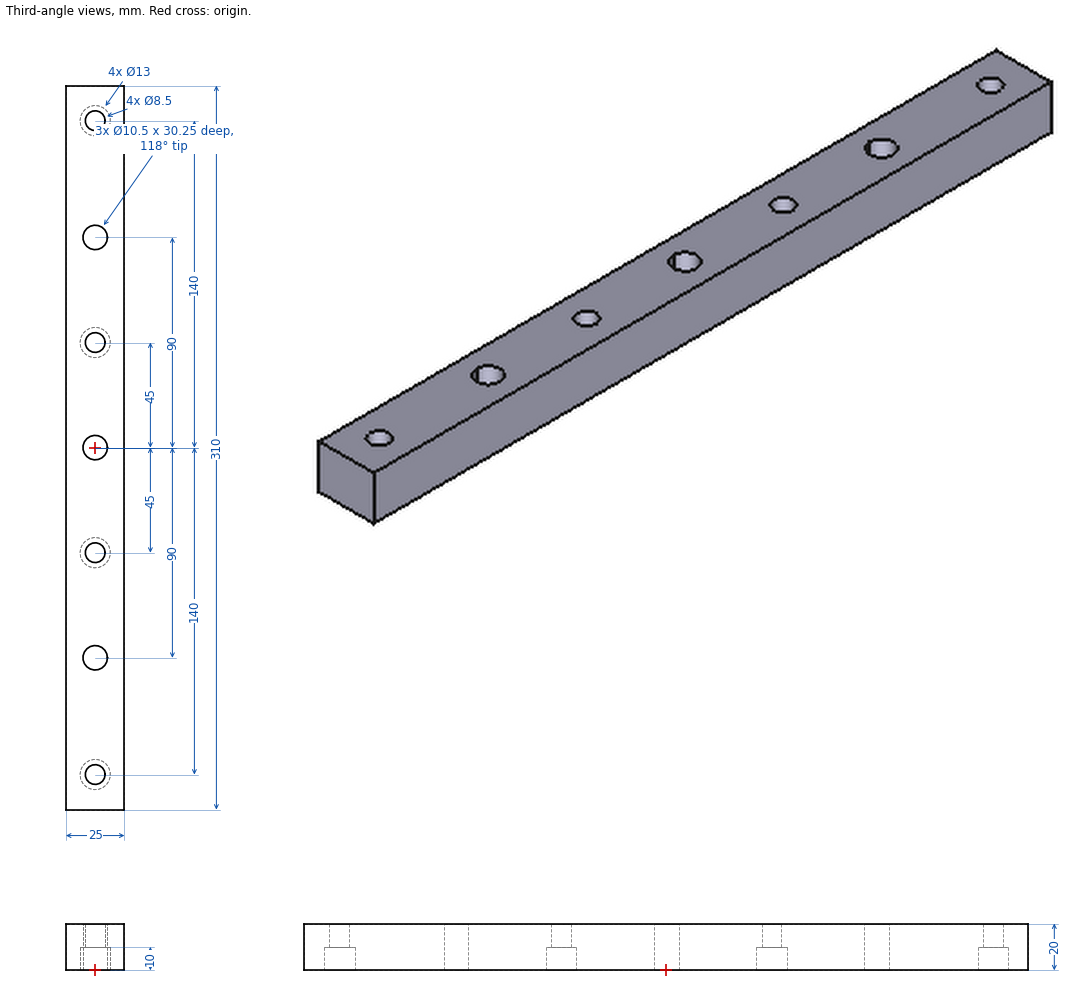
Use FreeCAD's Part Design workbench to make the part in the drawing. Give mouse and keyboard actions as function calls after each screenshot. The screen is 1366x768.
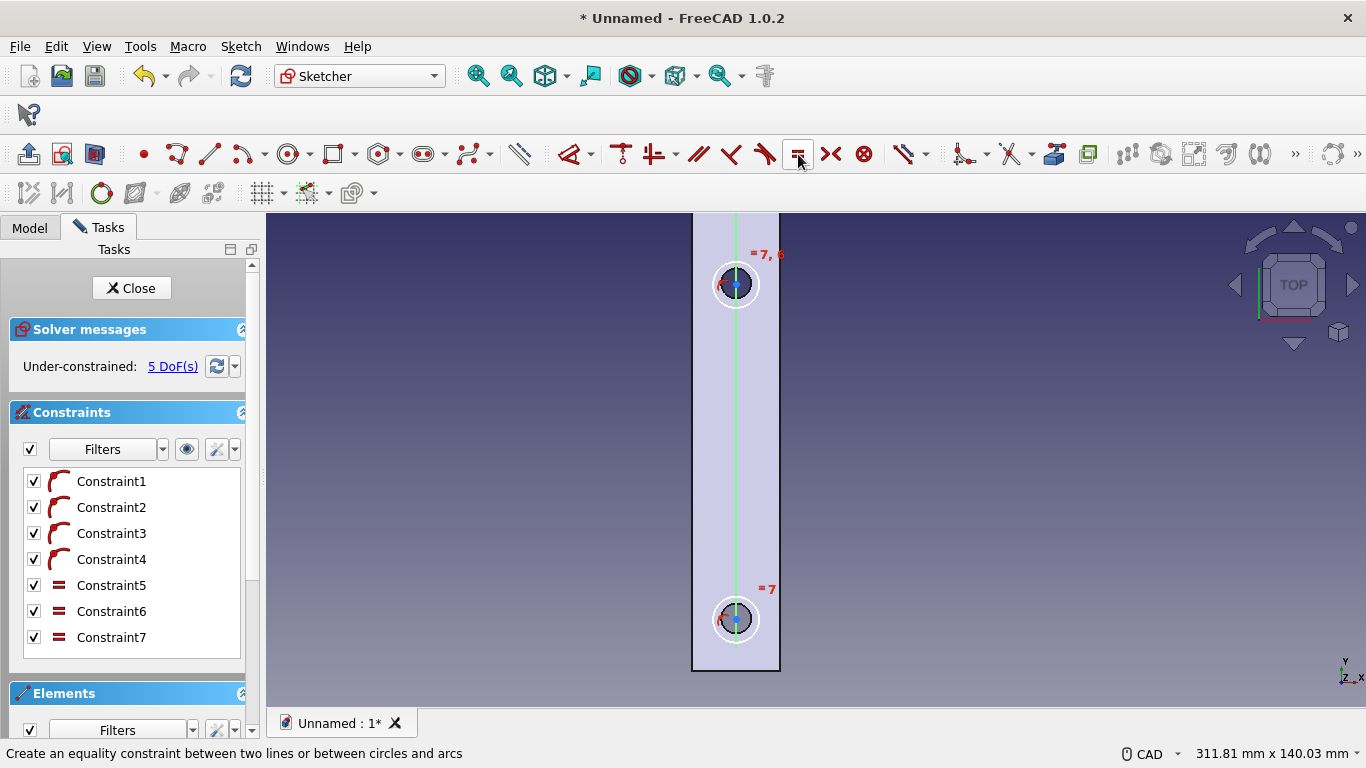
scroll(752, 605, down, 6)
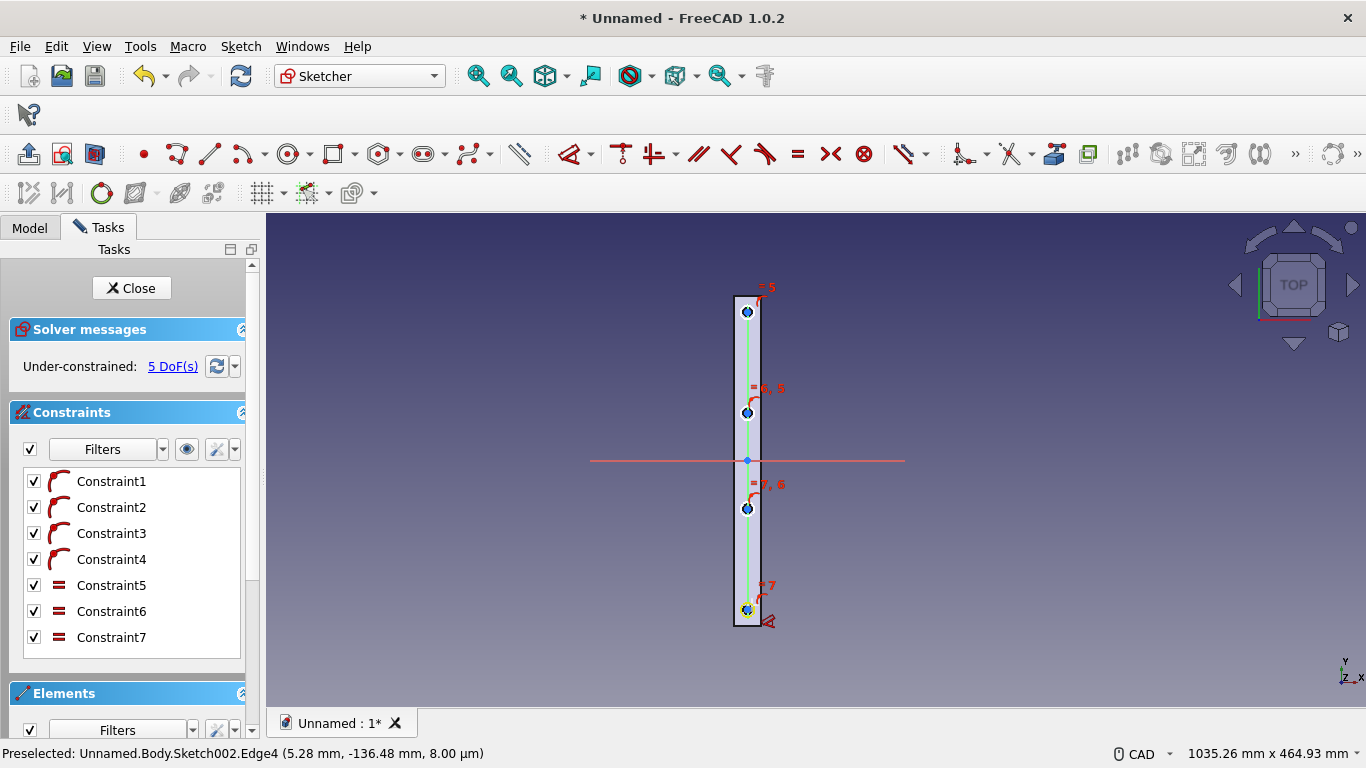
scroll(752, 308, up, 6)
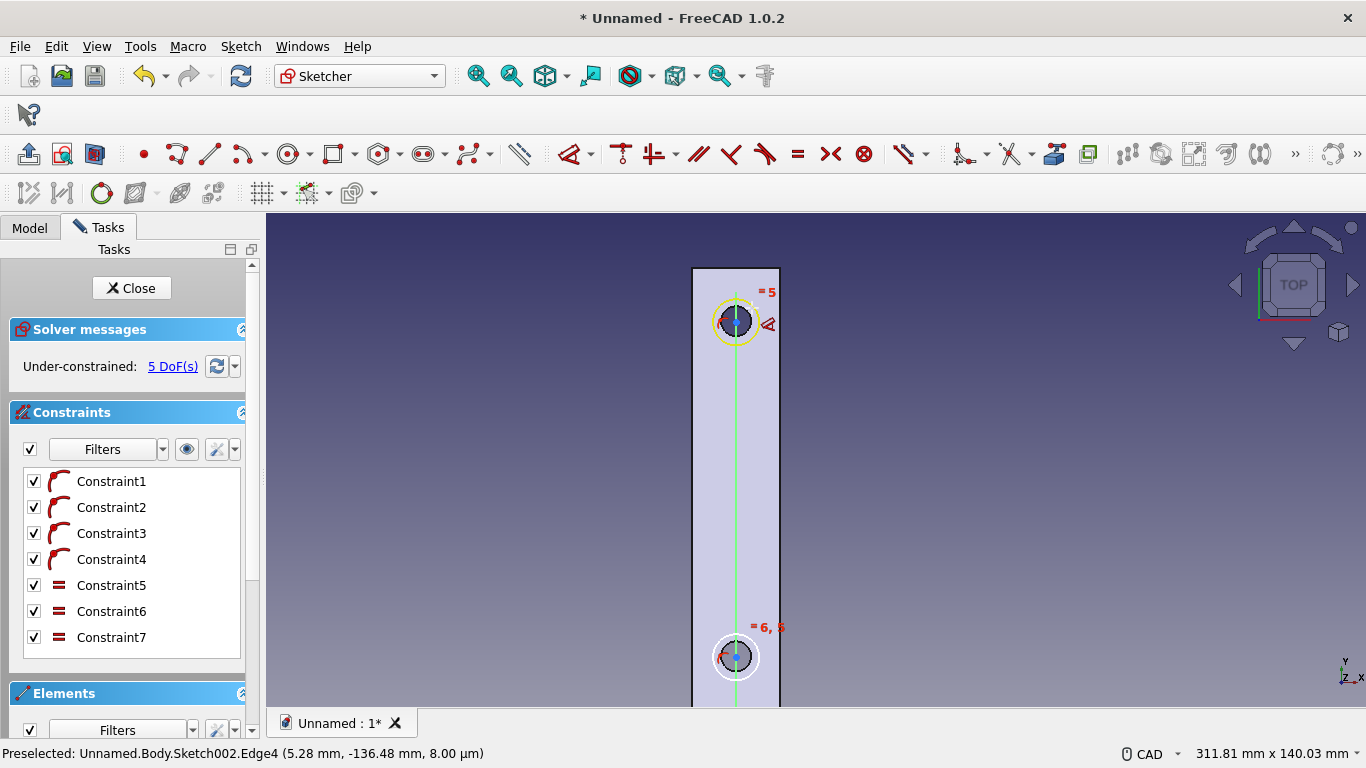
click(752, 306)
click(774, 283)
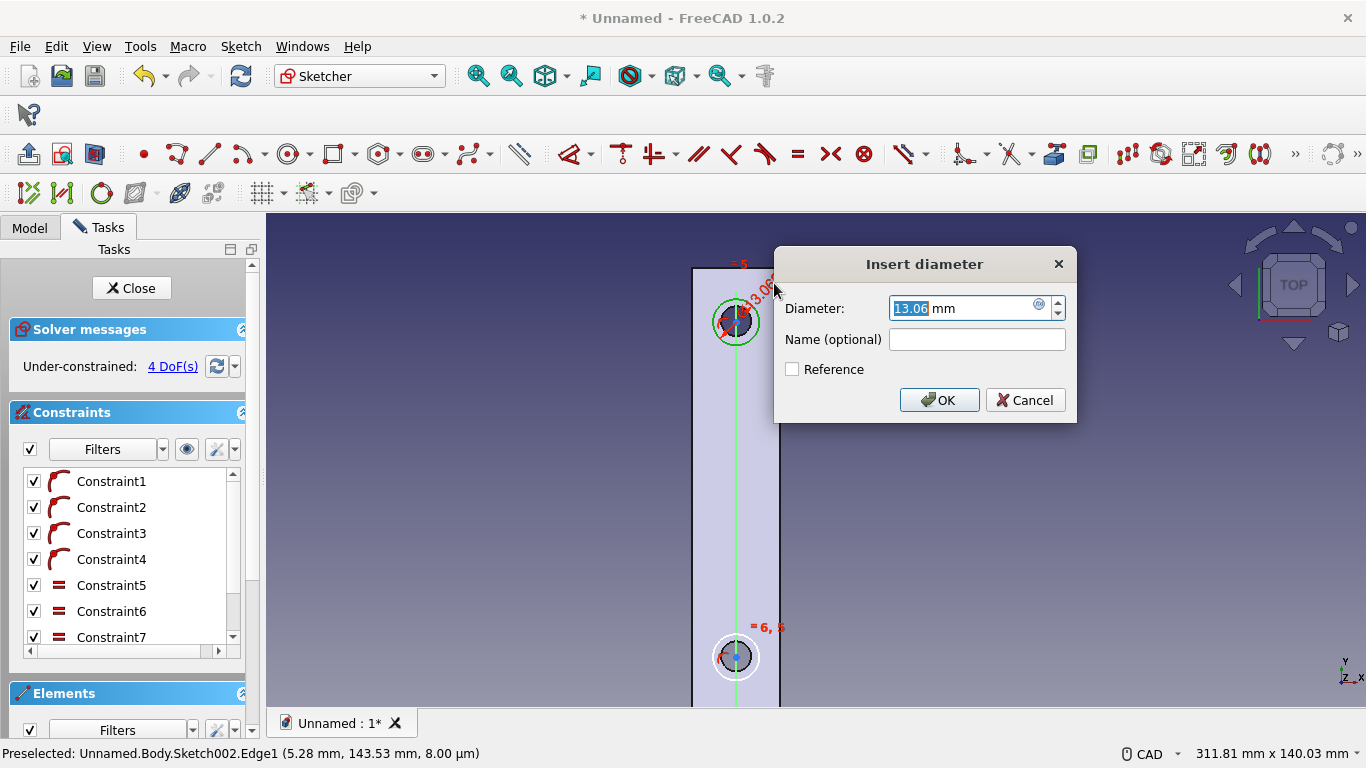
text(13)
key(Return)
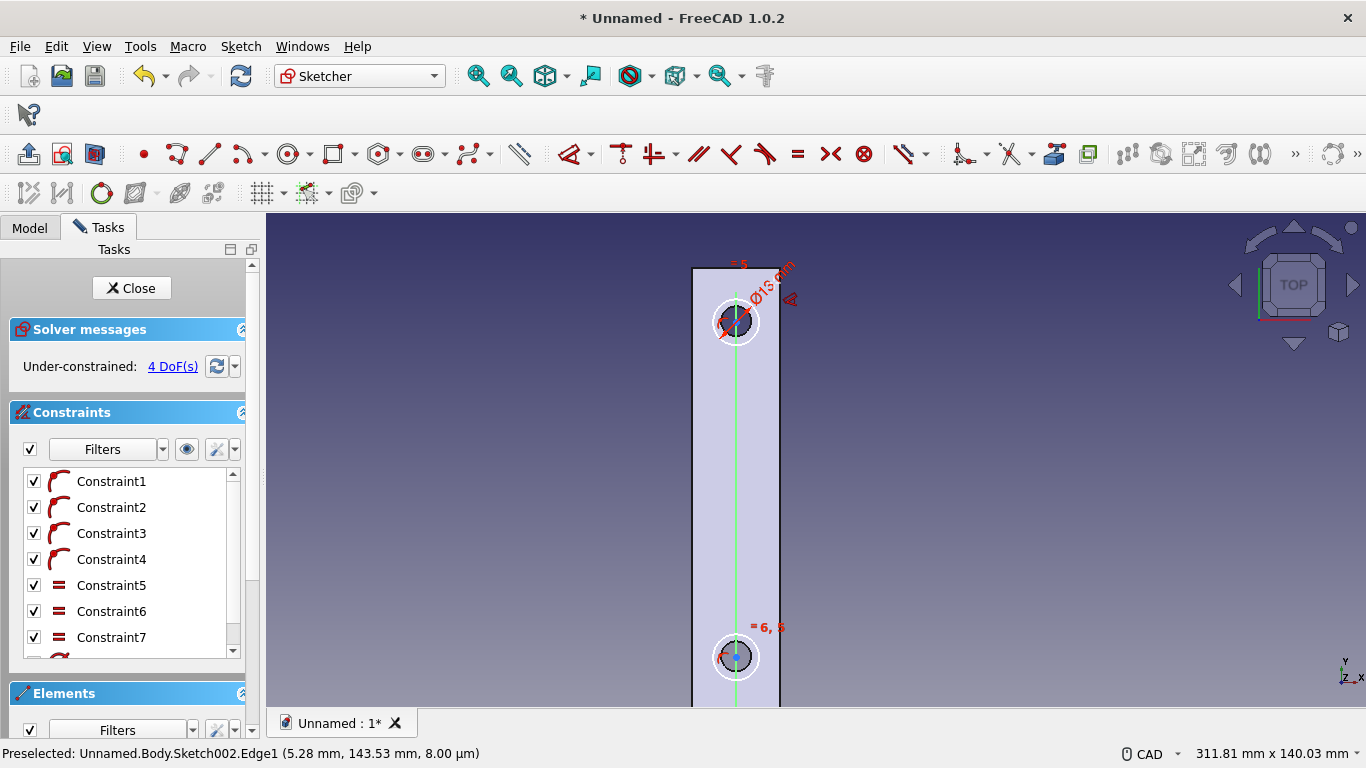
click(736, 657)
click(770, 673)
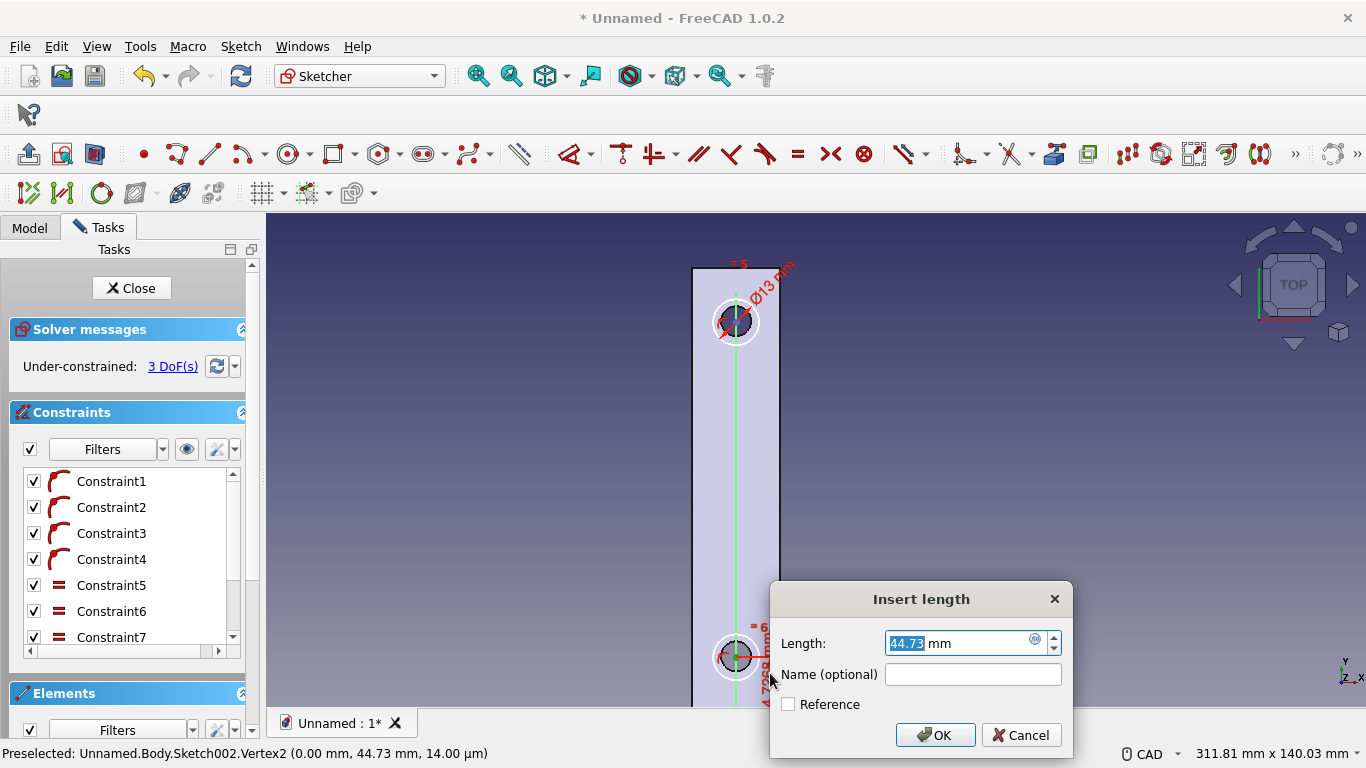
text(45)
key(Return)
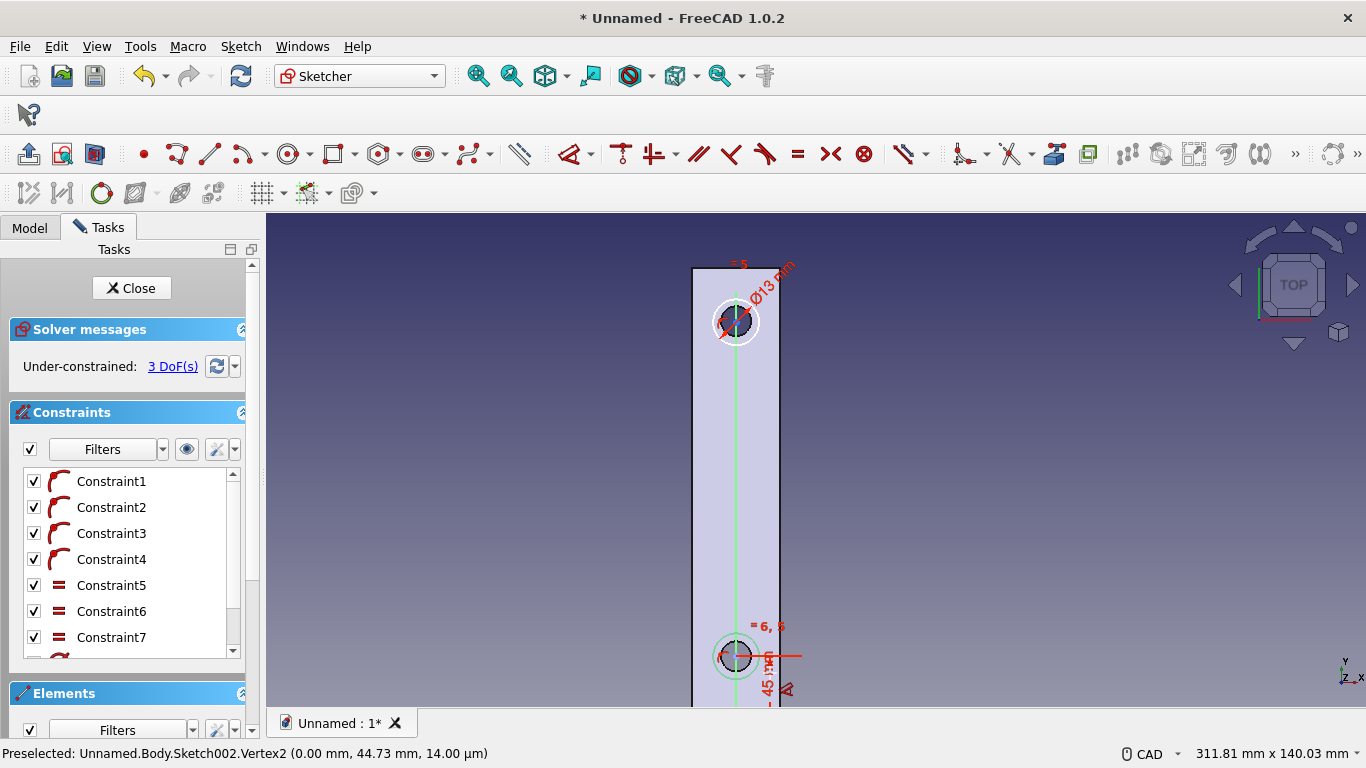
scroll(752, 307, down, 6)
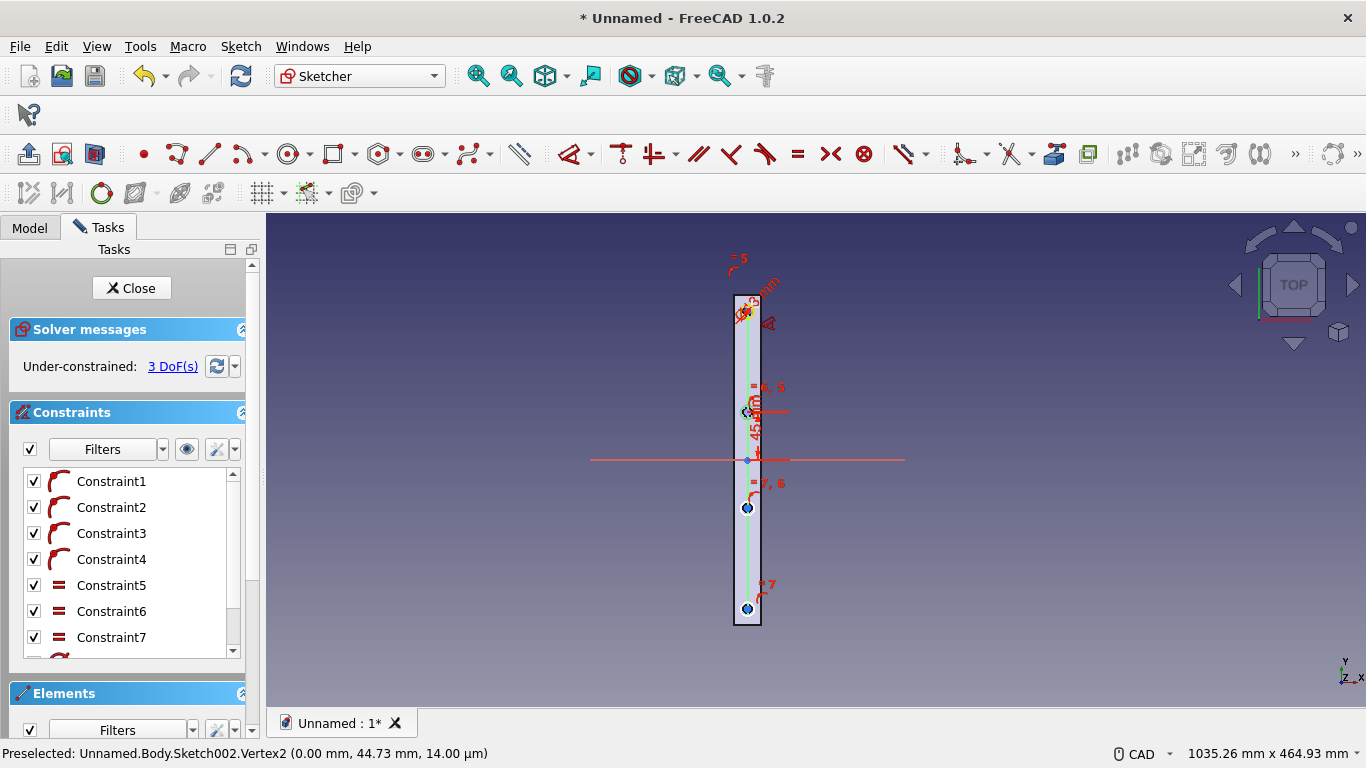
click(748, 508)
click(782, 484)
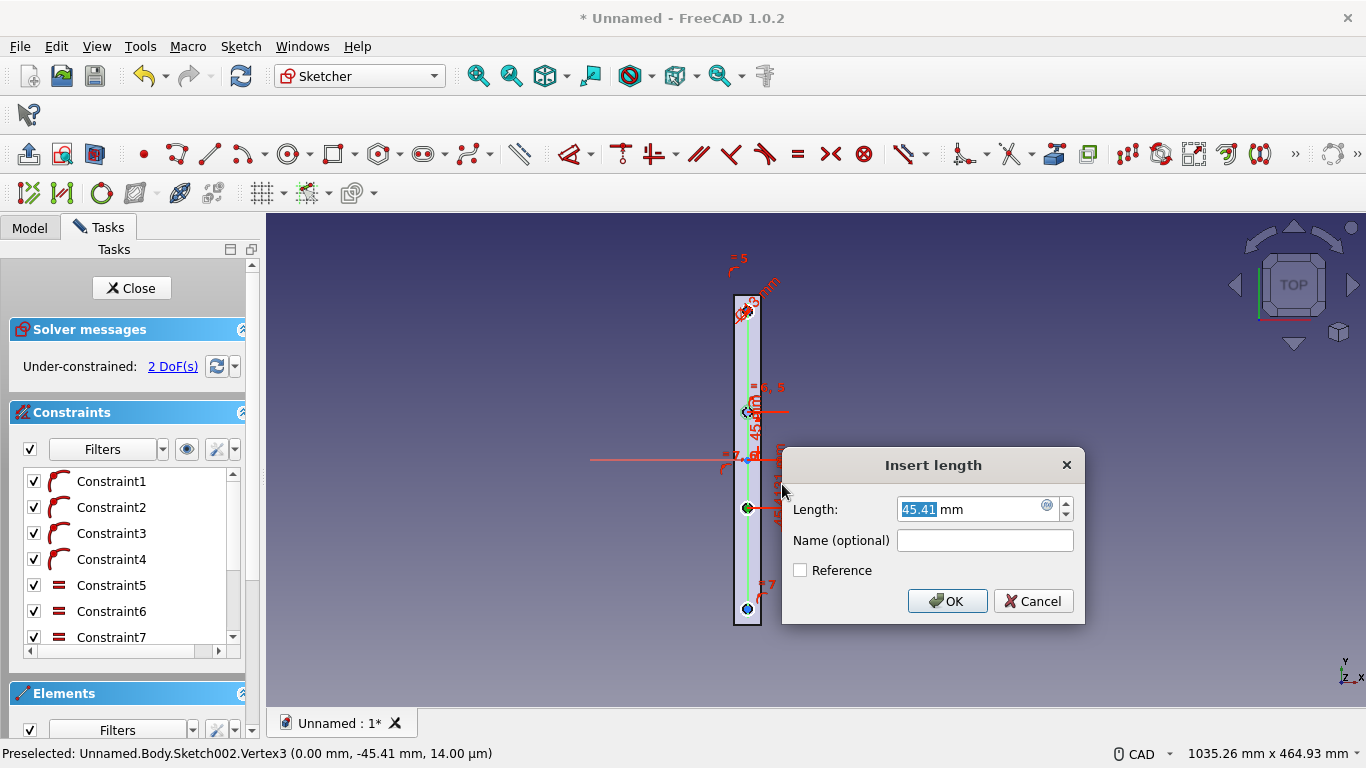
text(45)
key(Return)